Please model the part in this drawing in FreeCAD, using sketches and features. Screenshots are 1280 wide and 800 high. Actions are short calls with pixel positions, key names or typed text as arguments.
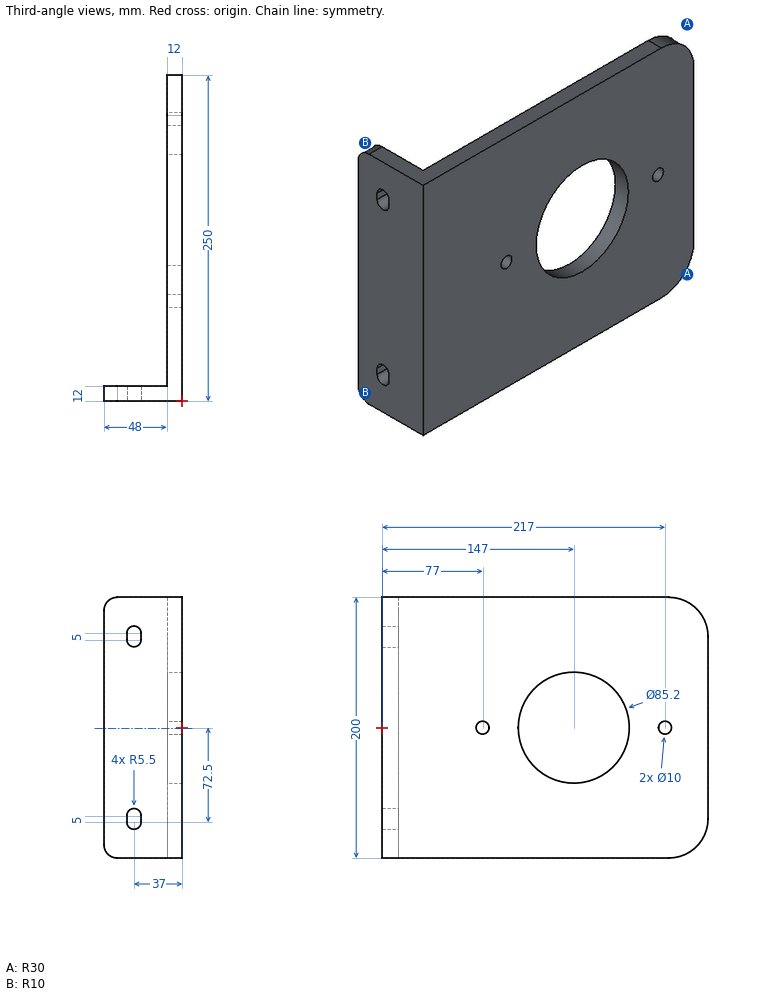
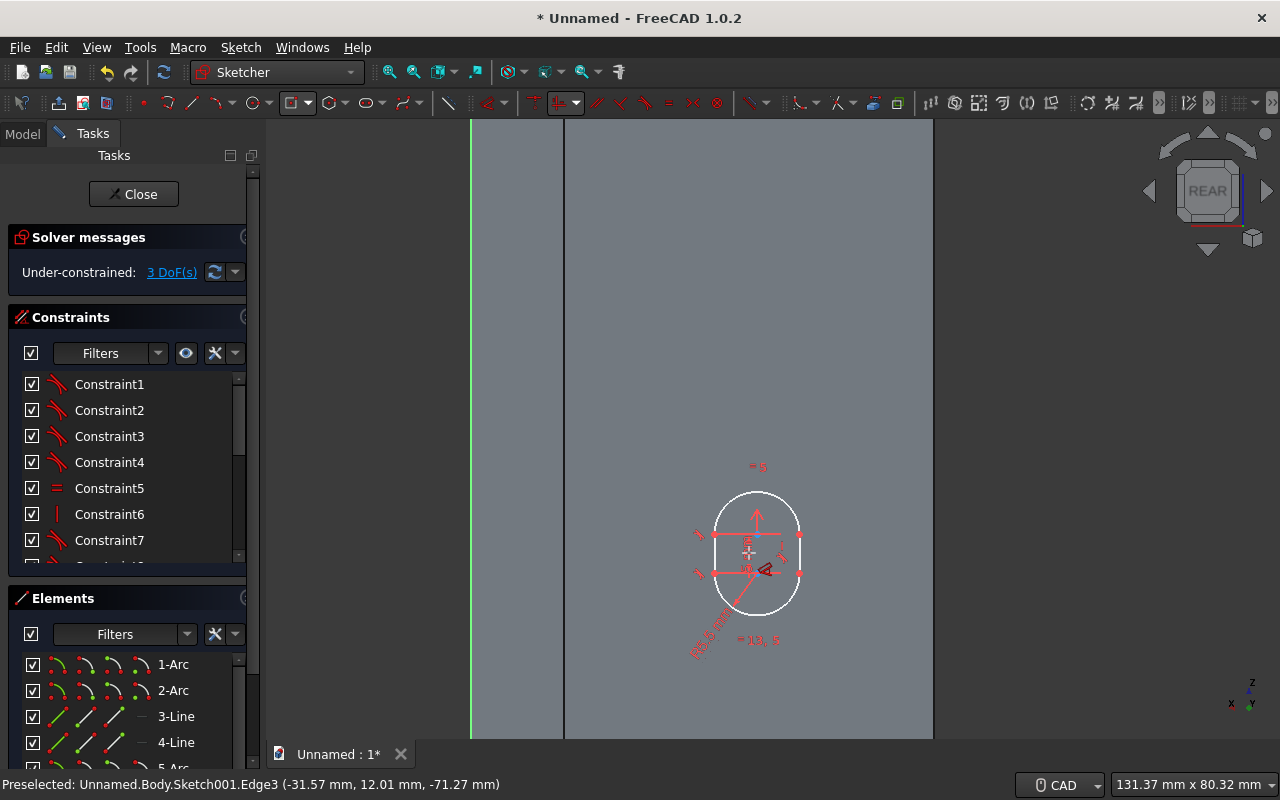
scroll(734, 609, down, 6)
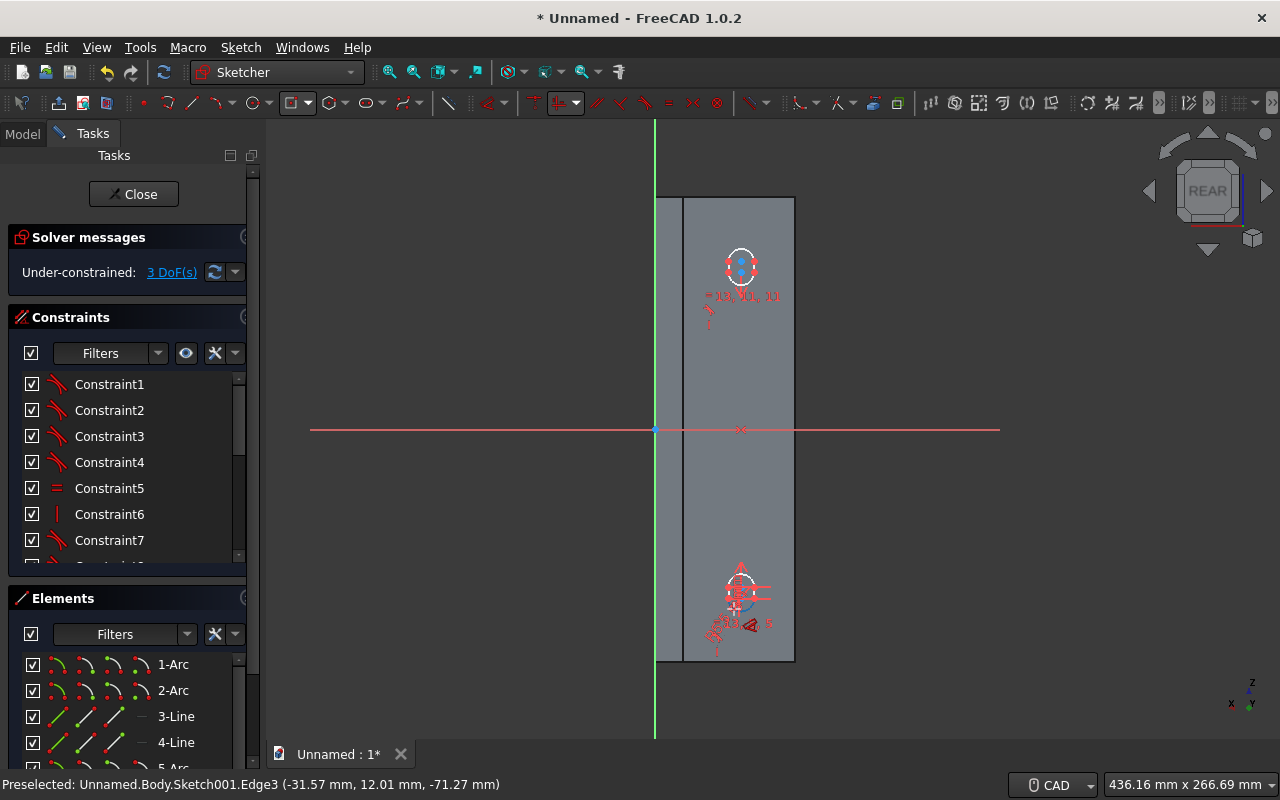
scroll(729, 269, up, 8)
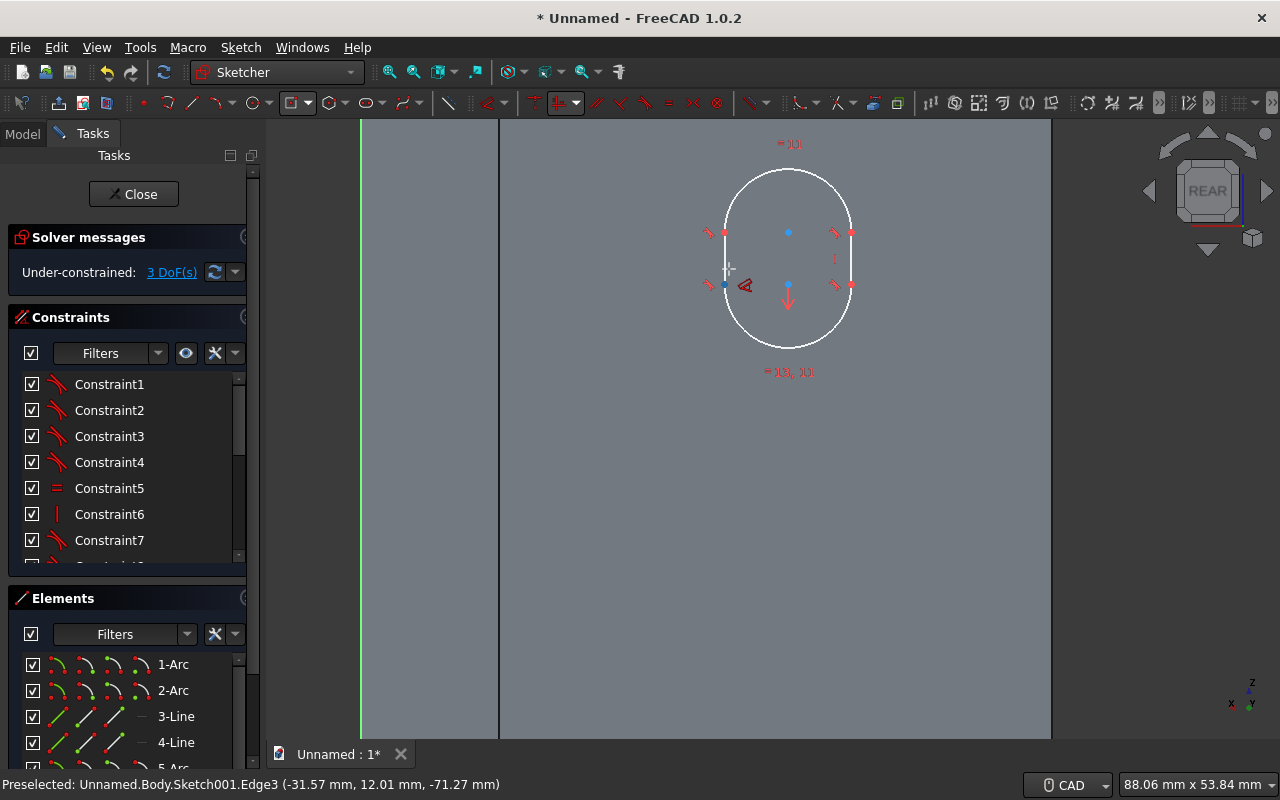
click(725, 269)
click(759, 259)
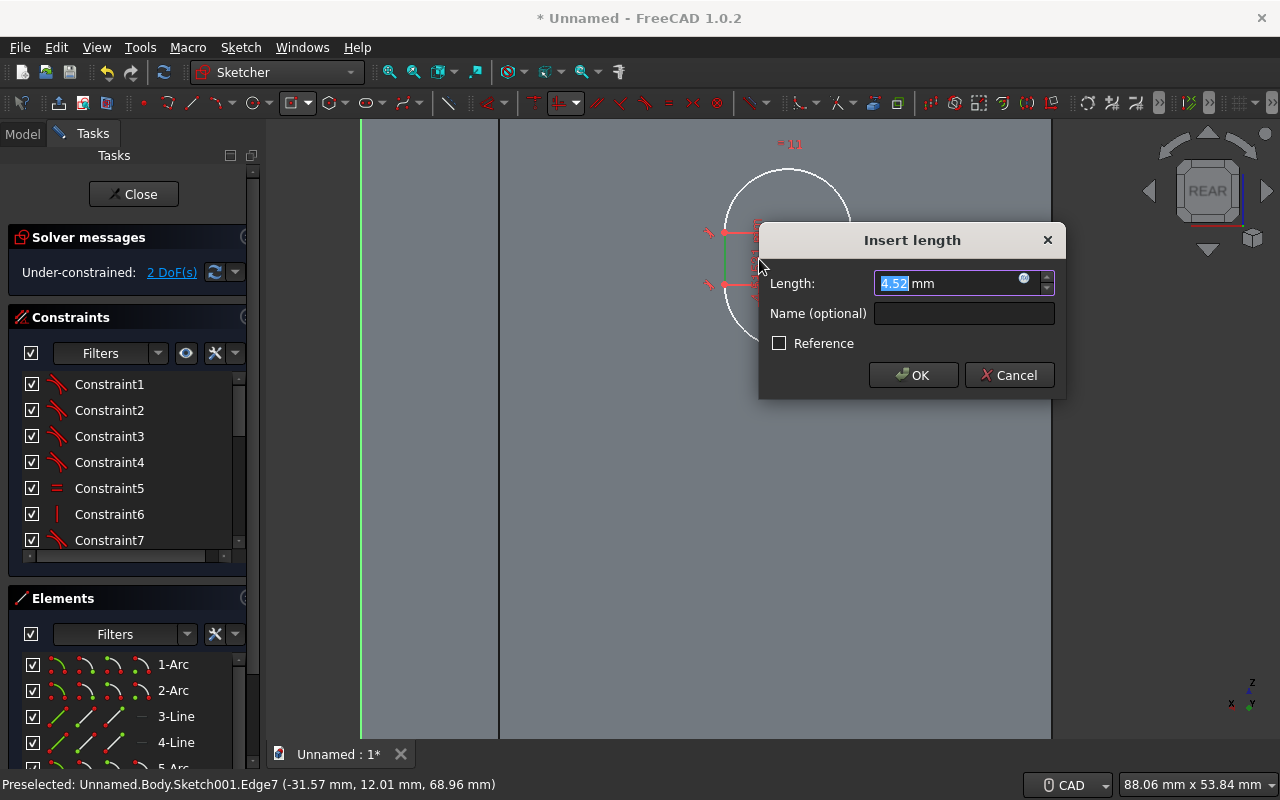
text(5)
key(Return)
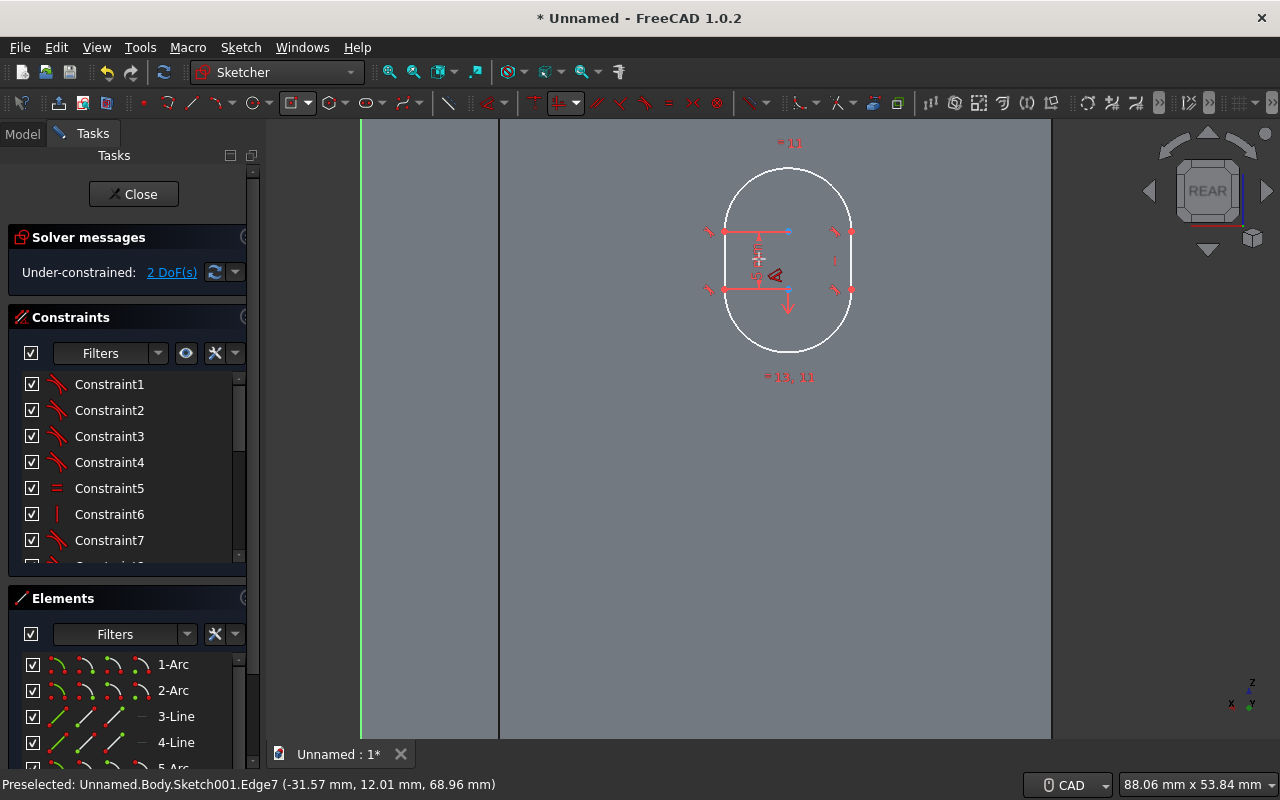
scroll(729, 268, down, 8)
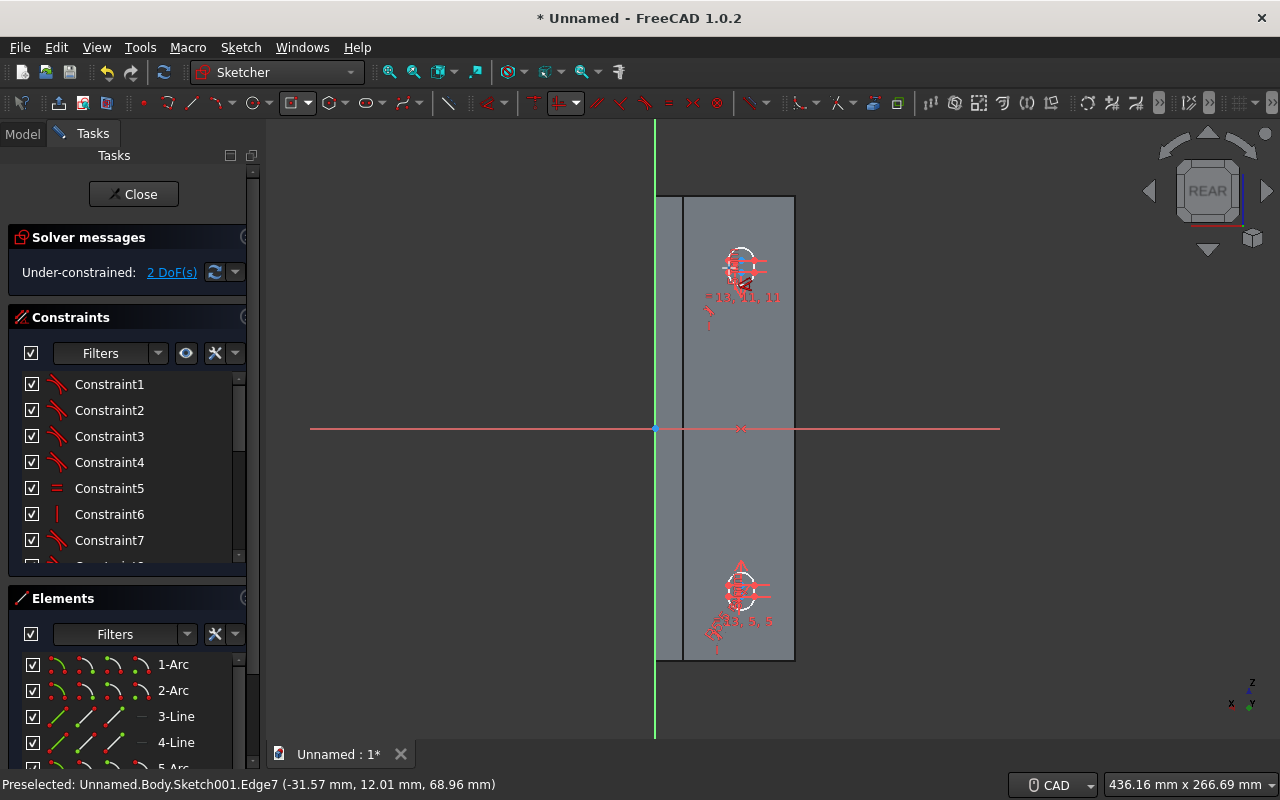
click(741, 597)
click(698, 395)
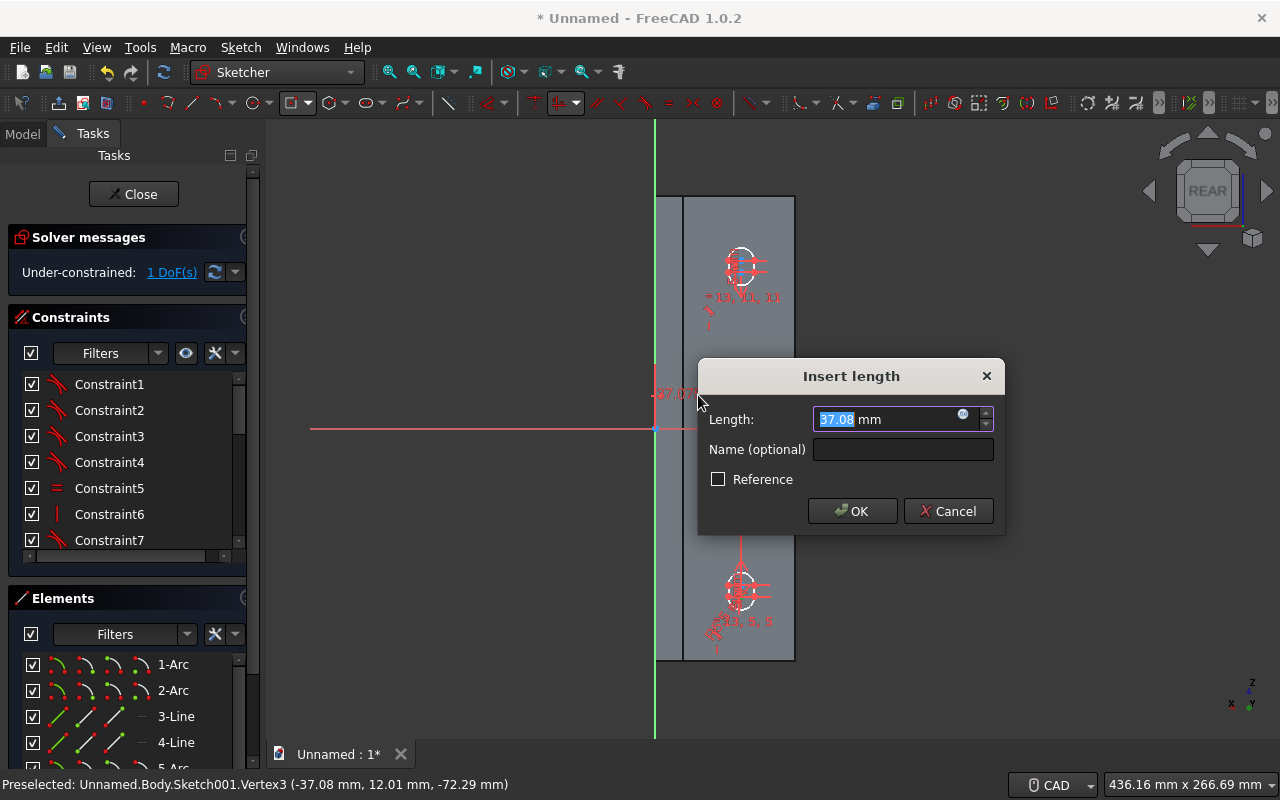
text(37)
key(Return)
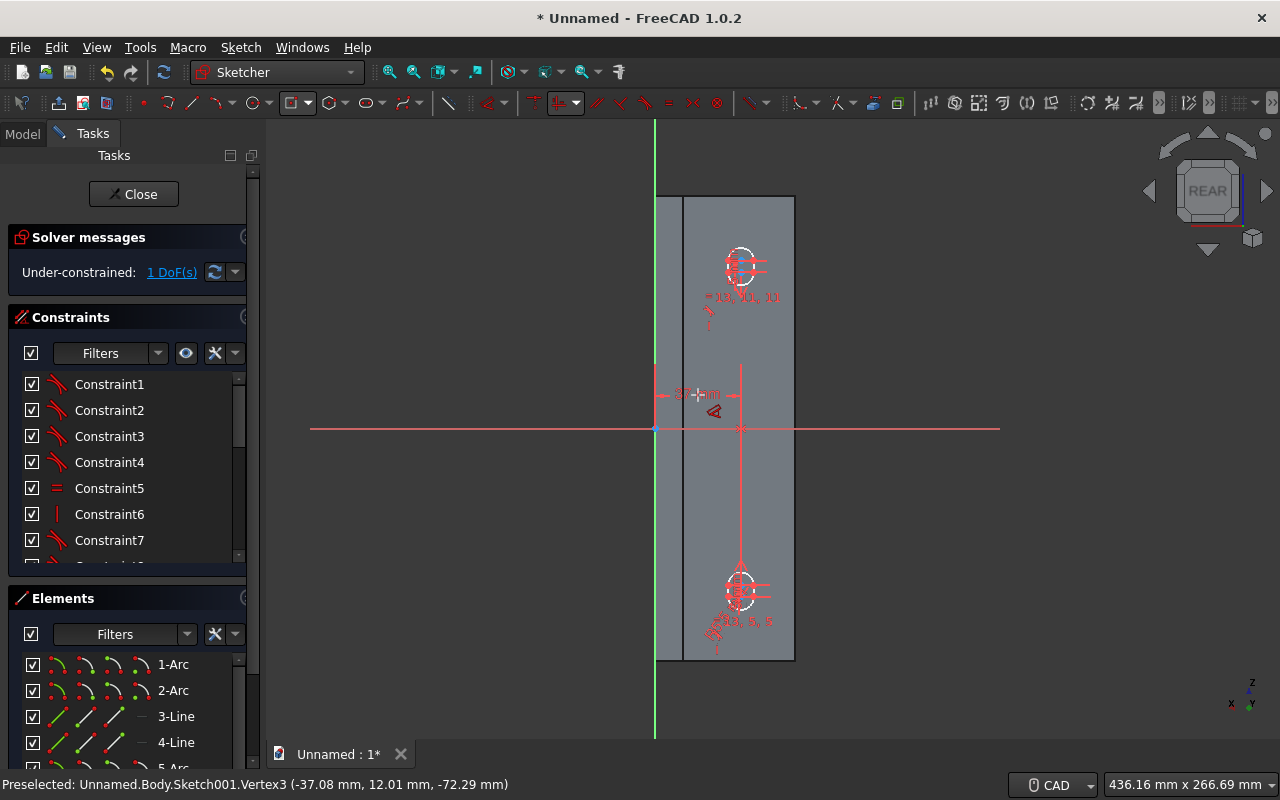
click(728, 597)
click(621, 513)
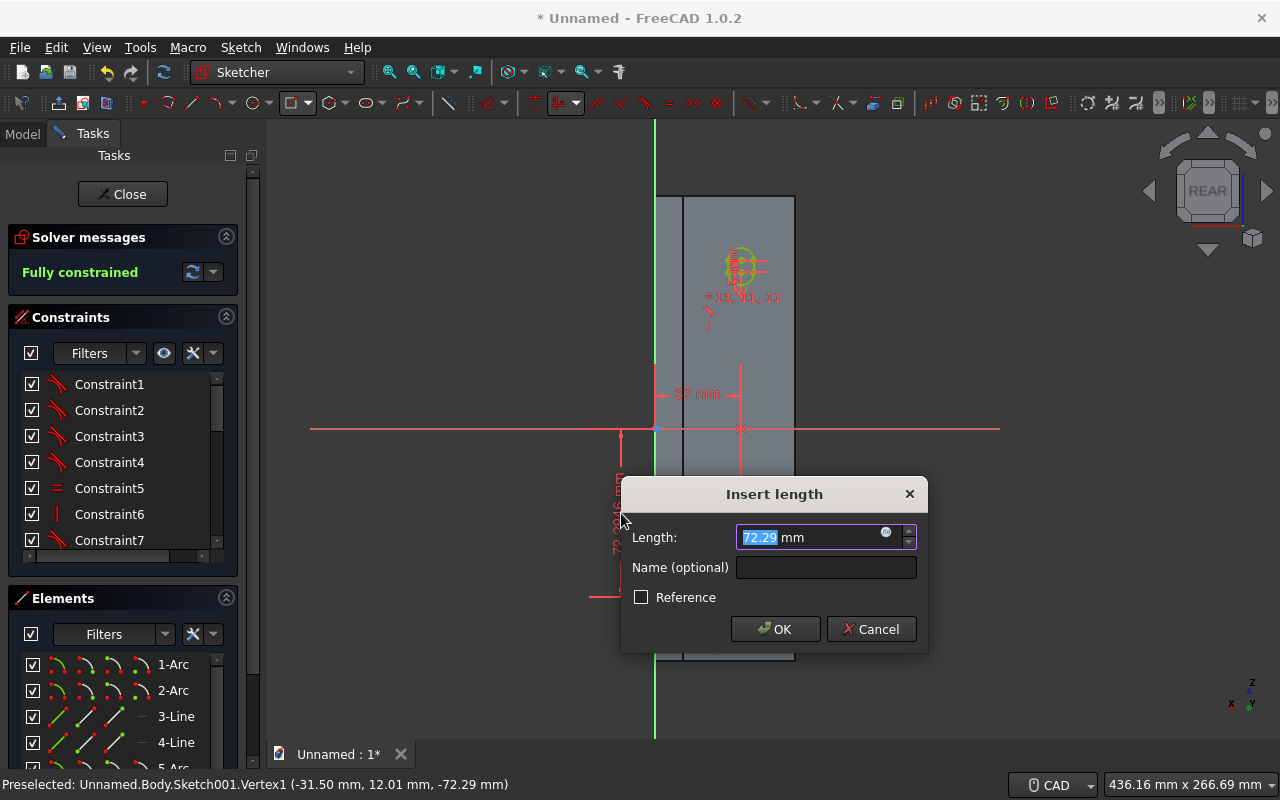
text(72.5)
key(Return)
key(Escape)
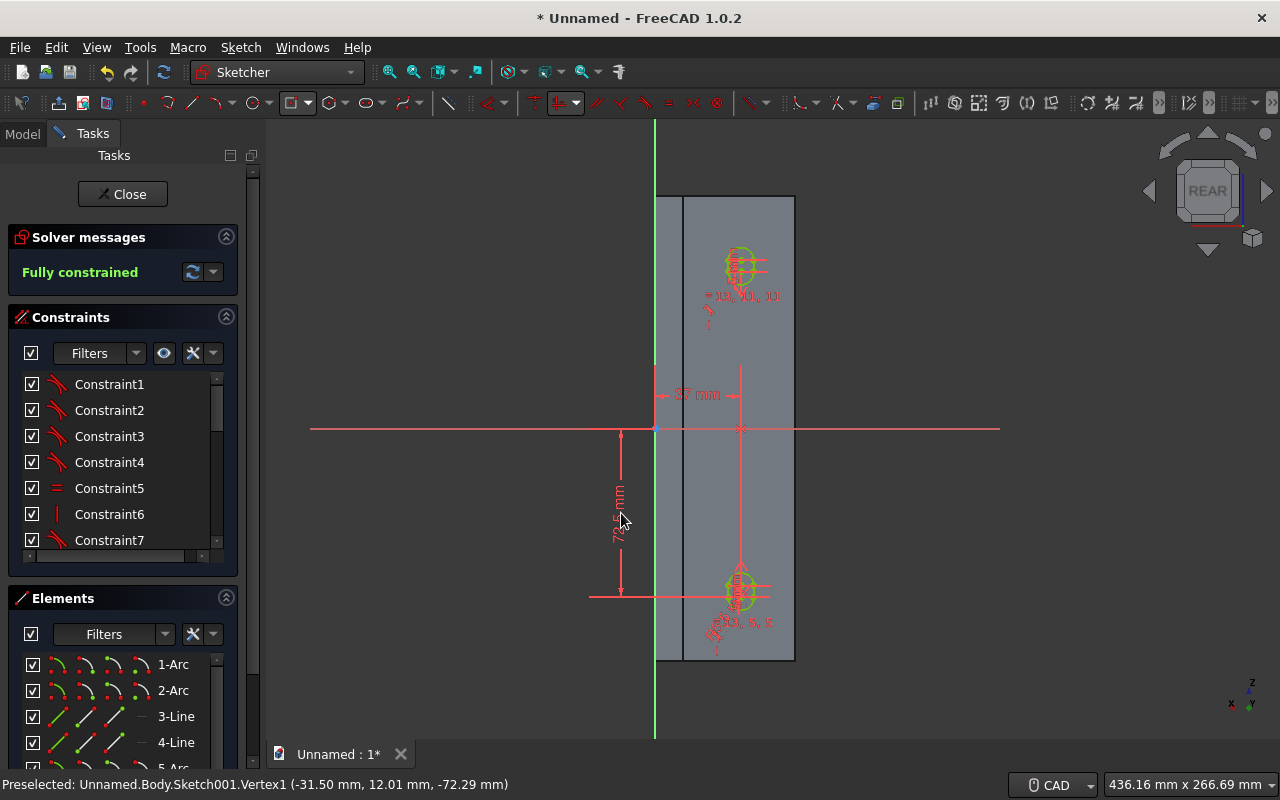
click(123, 194)